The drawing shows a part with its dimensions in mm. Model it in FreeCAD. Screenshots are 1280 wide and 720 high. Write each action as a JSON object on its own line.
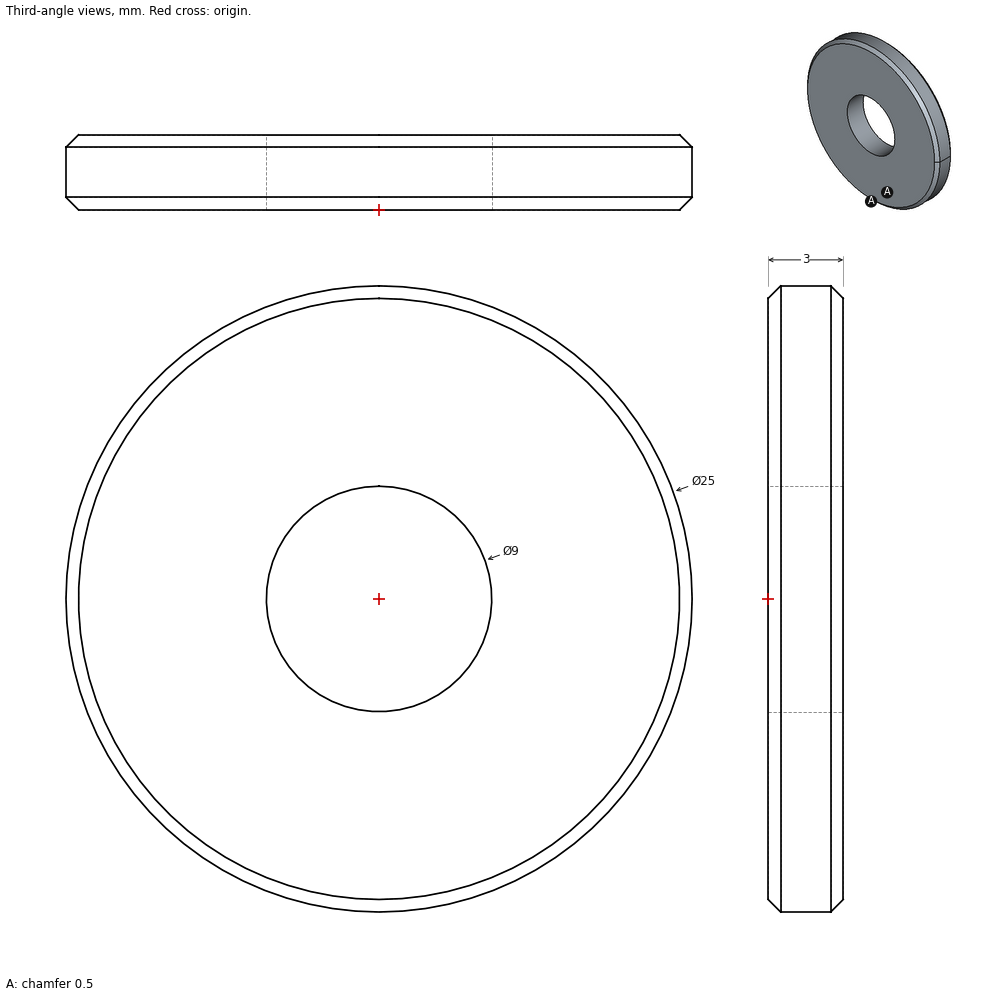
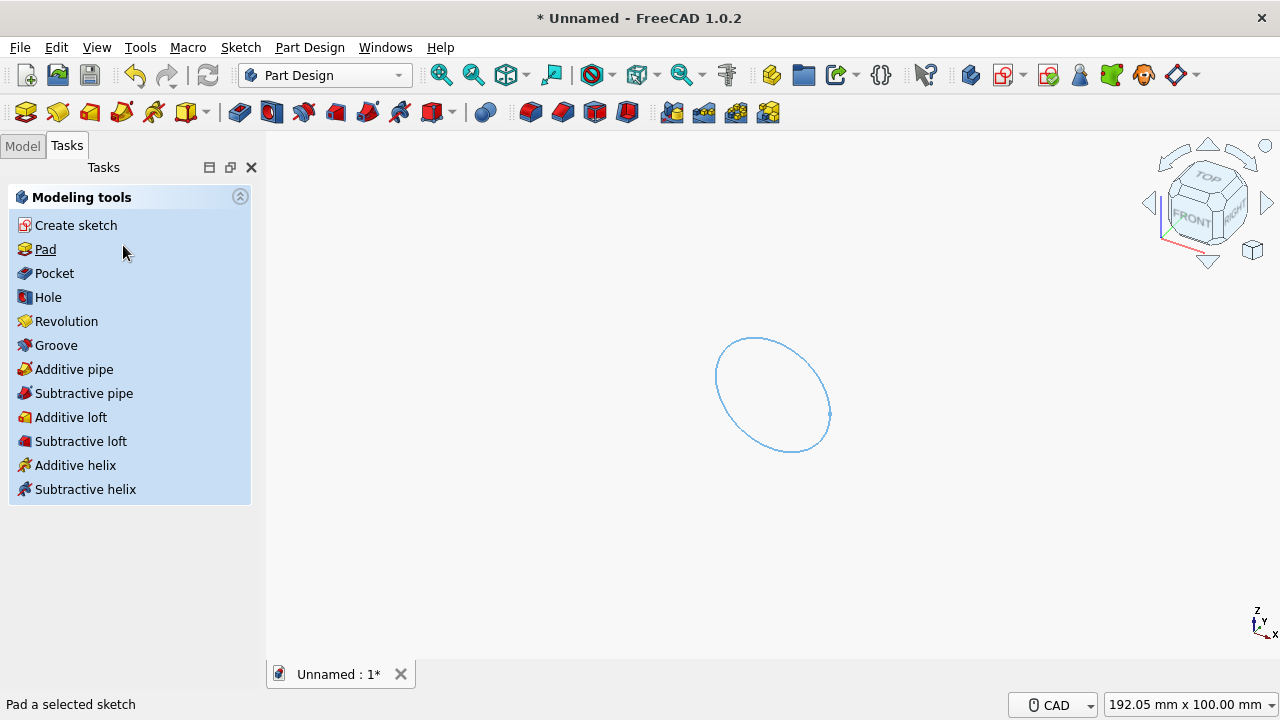
{"action": "left_click", "coordinate": [26, 112]}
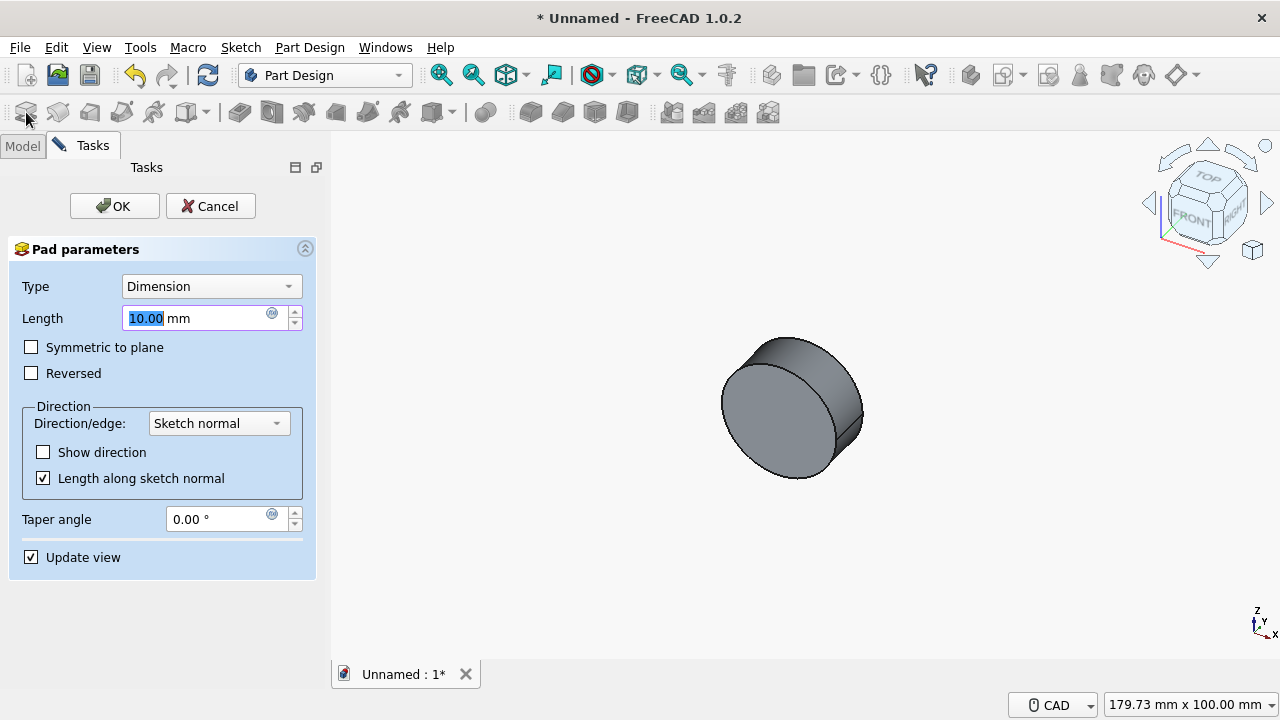
{"action": "type", "text": "3"}
{"action": "key", "text": "Tab"}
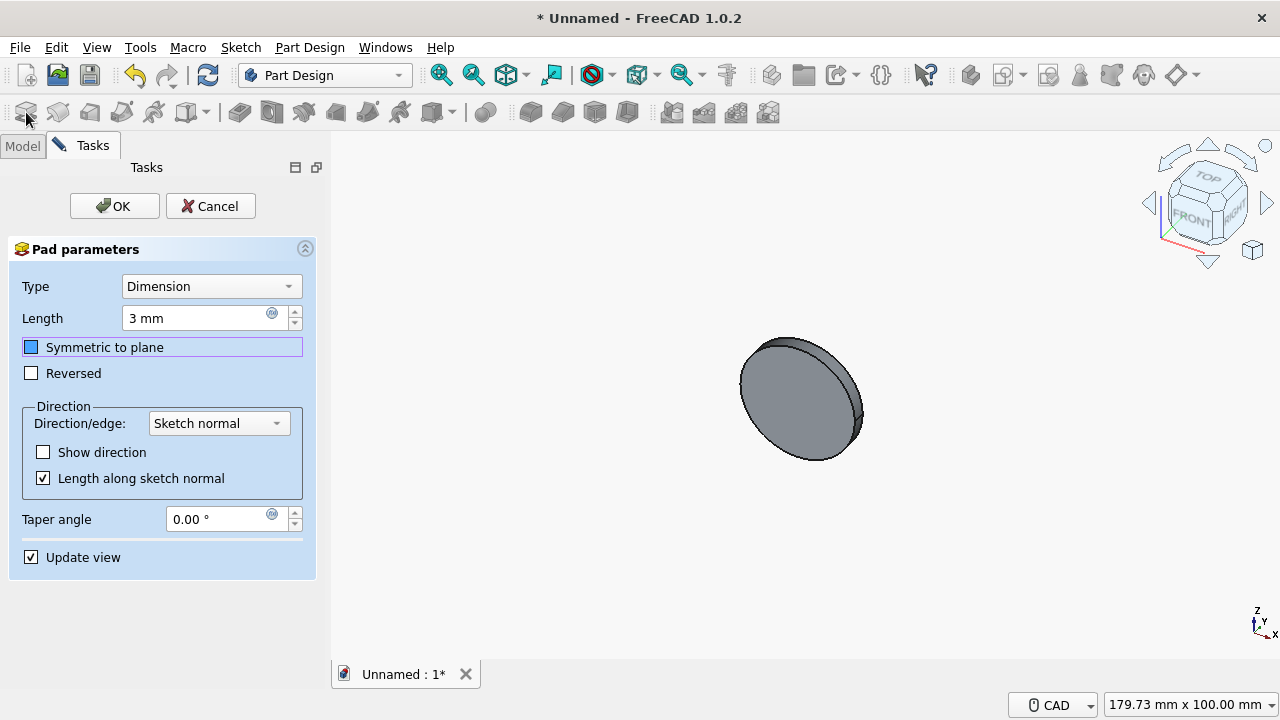
{"action": "left_click", "coordinate": [30, 373]}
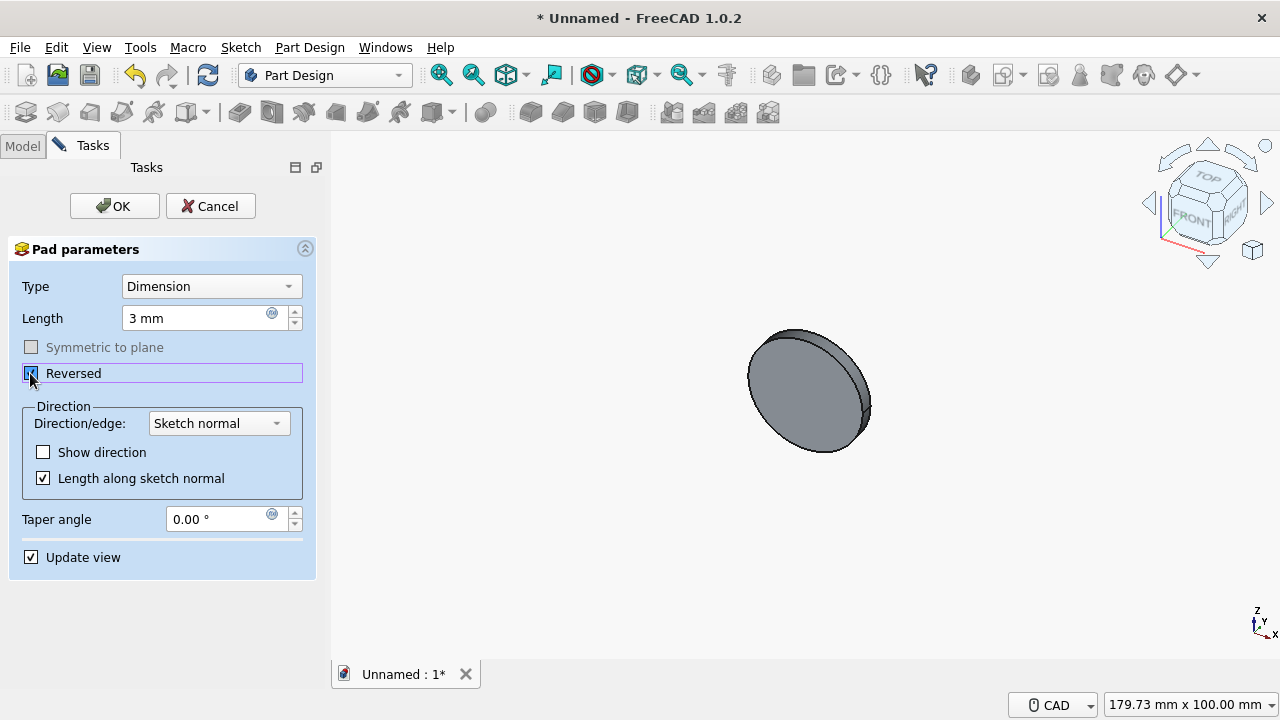
{"action": "left_click", "coordinate": [115, 206]}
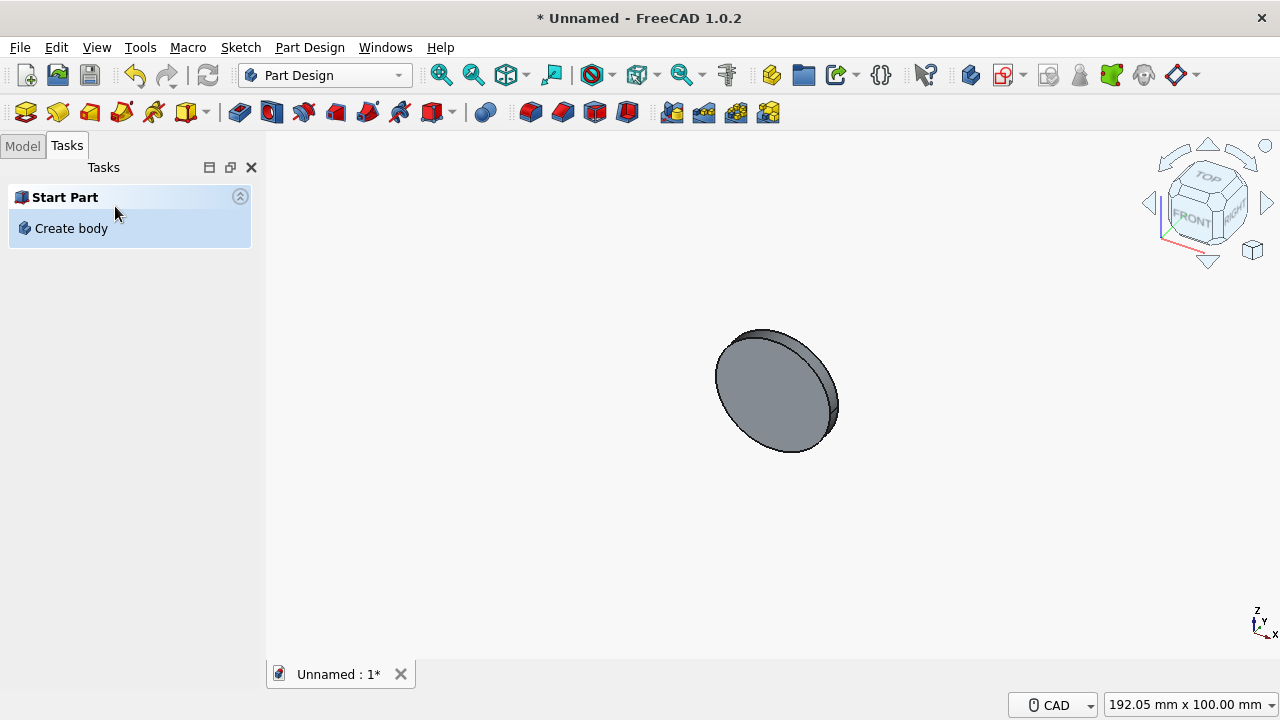
{"action": "left_click", "coordinate": [442, 76]}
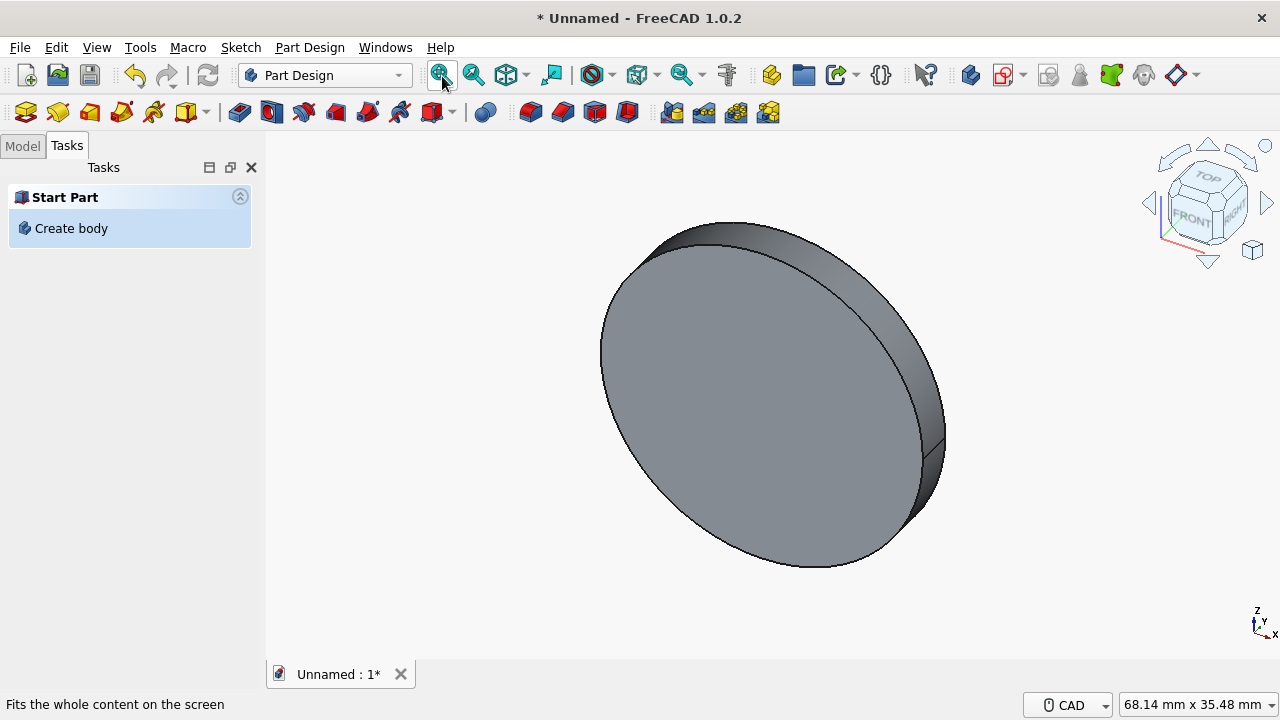
{"action": "key", "text": "4"}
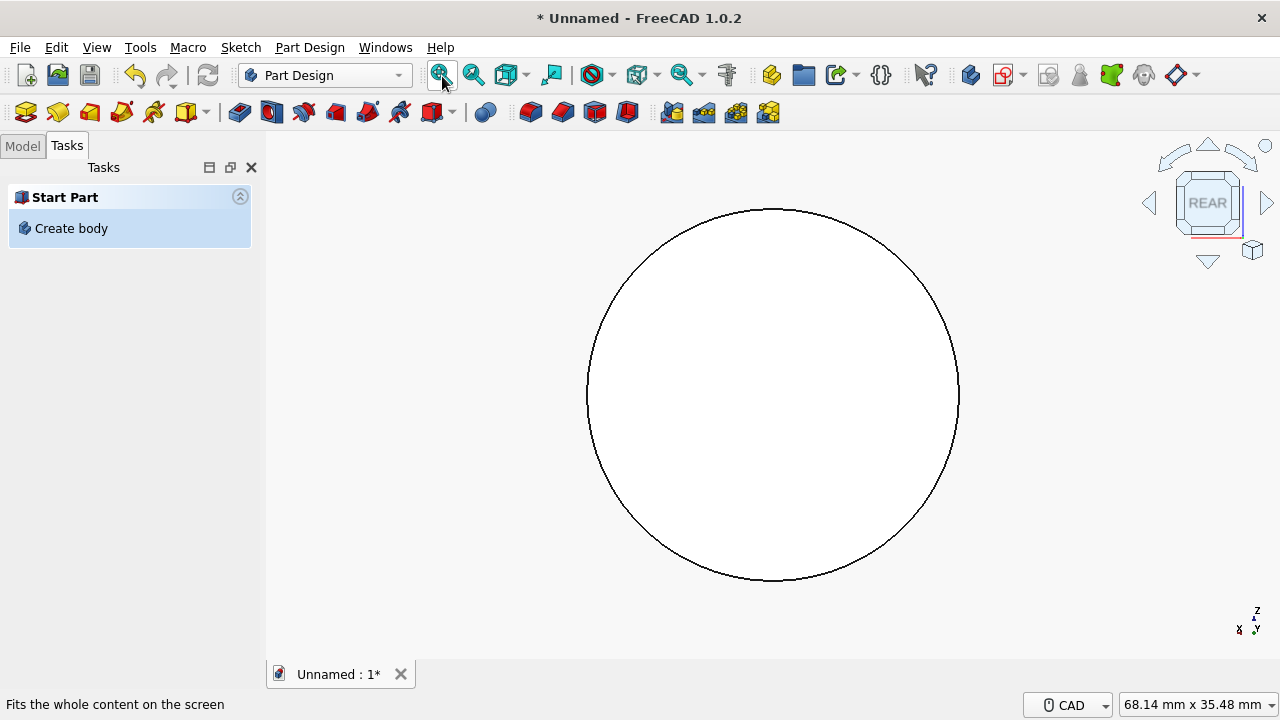
{"action": "left_click", "coordinate": [773, 394]}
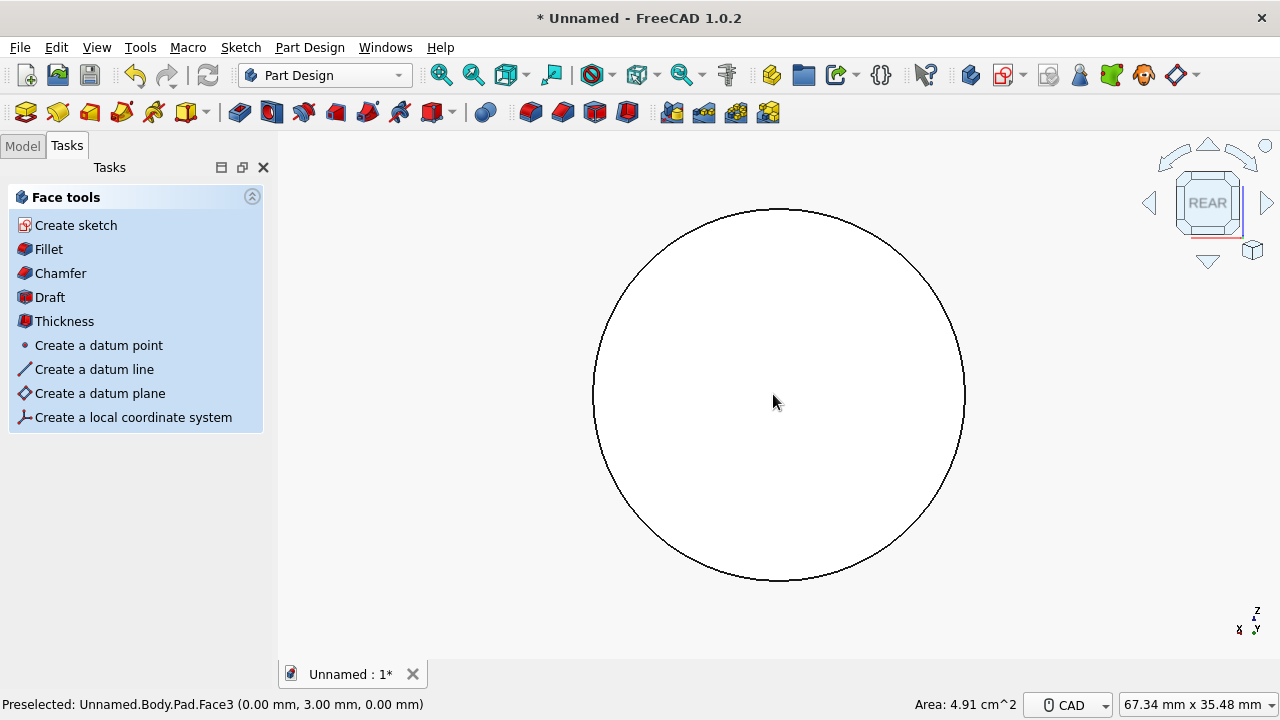
{"action": "left_click", "coordinate": [1004, 76]}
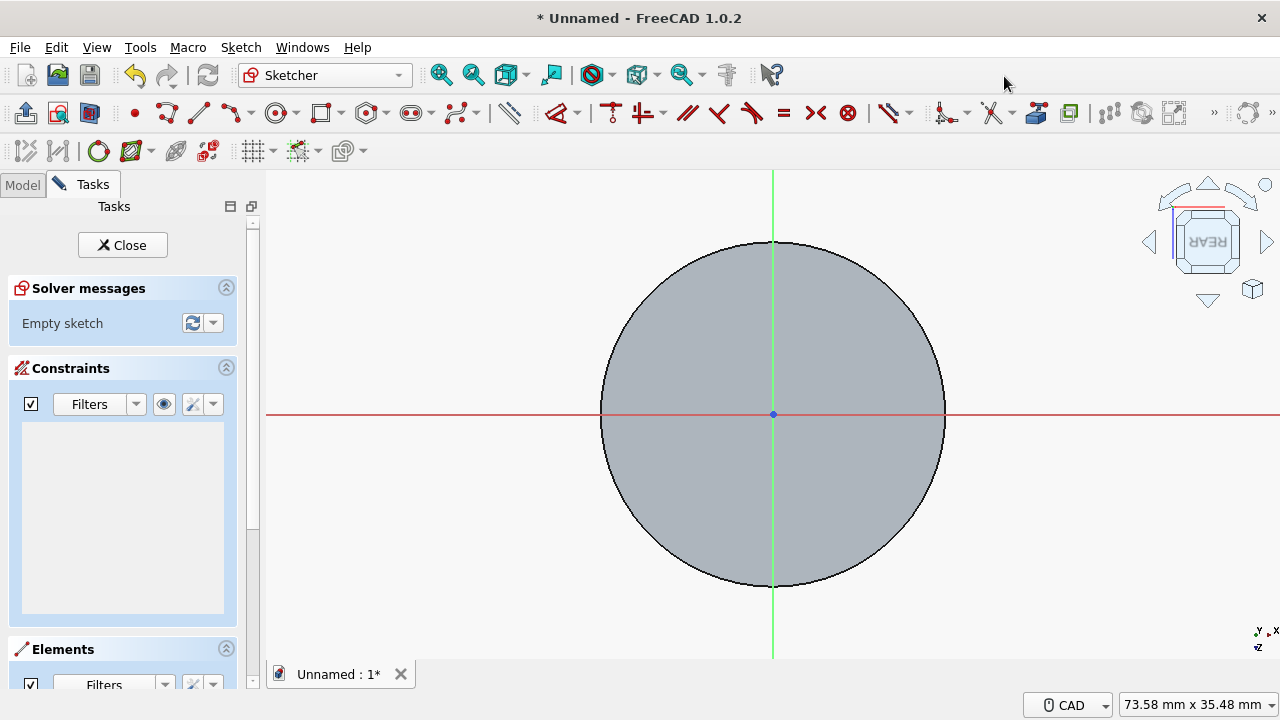
{"action": "scroll", "coordinate": [813, 415], "scroll_direction": "up", "scroll_amount": 5}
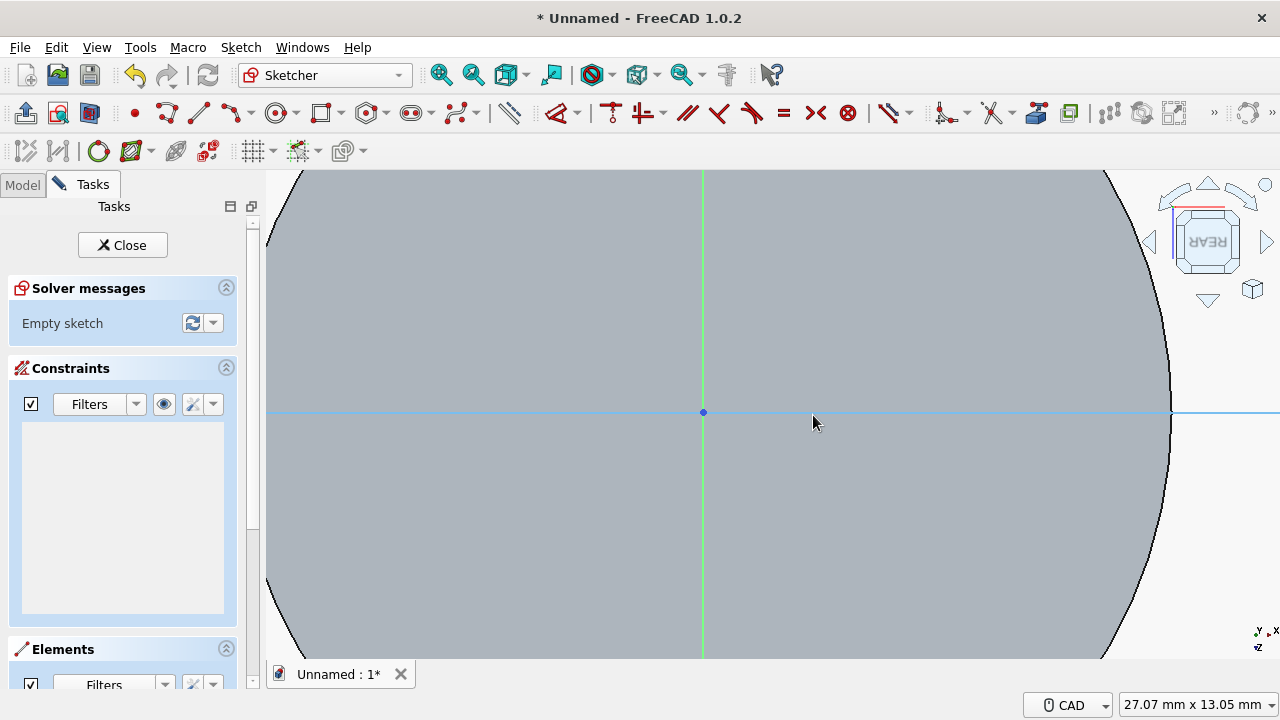
{"action": "left_click", "coordinate": [276, 114]}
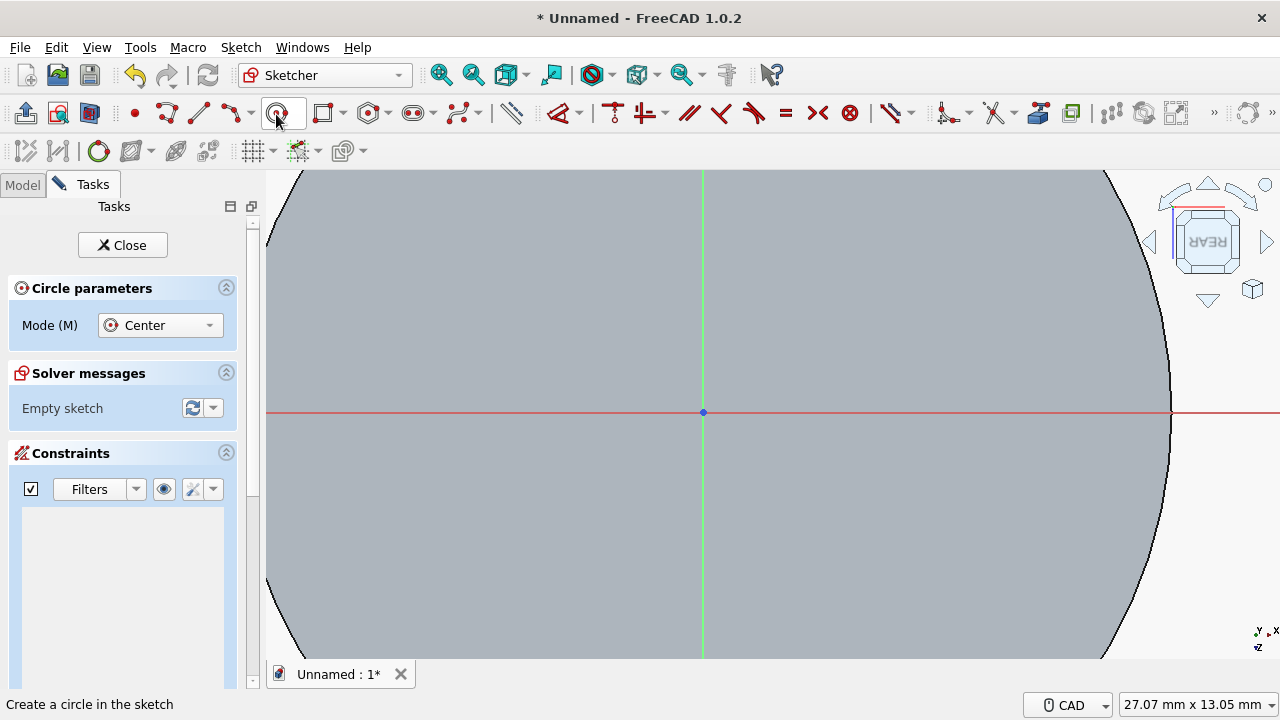
{"action": "left_click", "coordinate": [703, 413]}
{"action": "left_click", "coordinate": [823, 294]}
{"action": "key", "text": "Escape"}